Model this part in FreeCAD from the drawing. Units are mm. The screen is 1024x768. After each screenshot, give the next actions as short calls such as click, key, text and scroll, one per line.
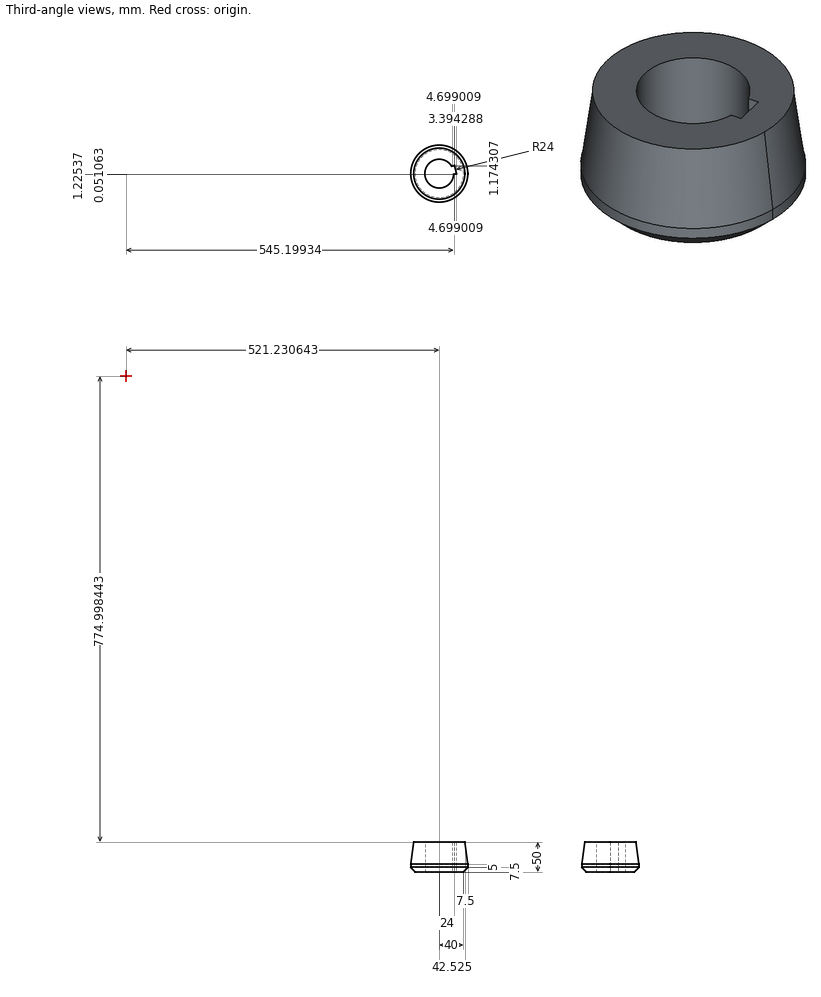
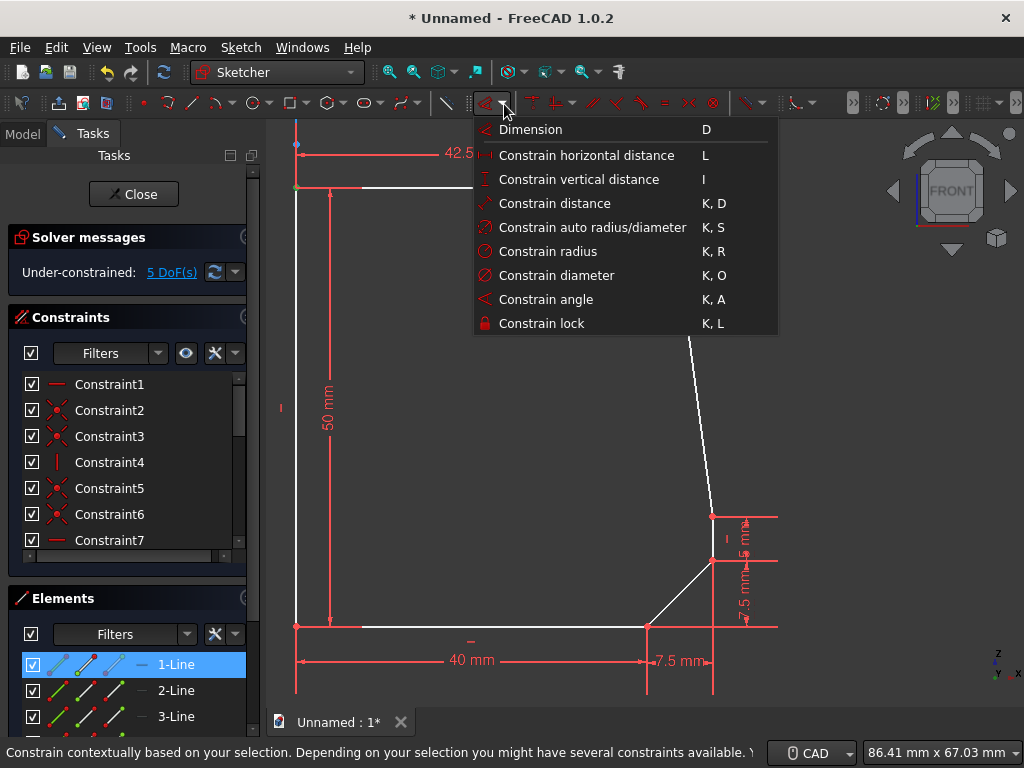
click(626, 155)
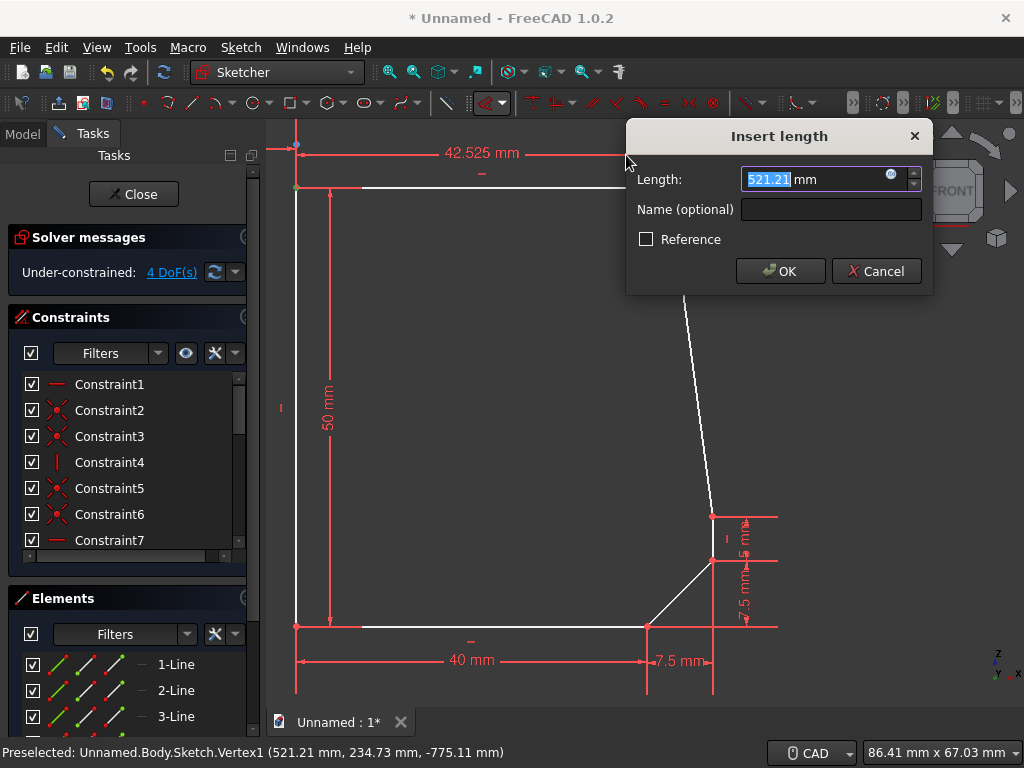
text(521.230643)
key(Return)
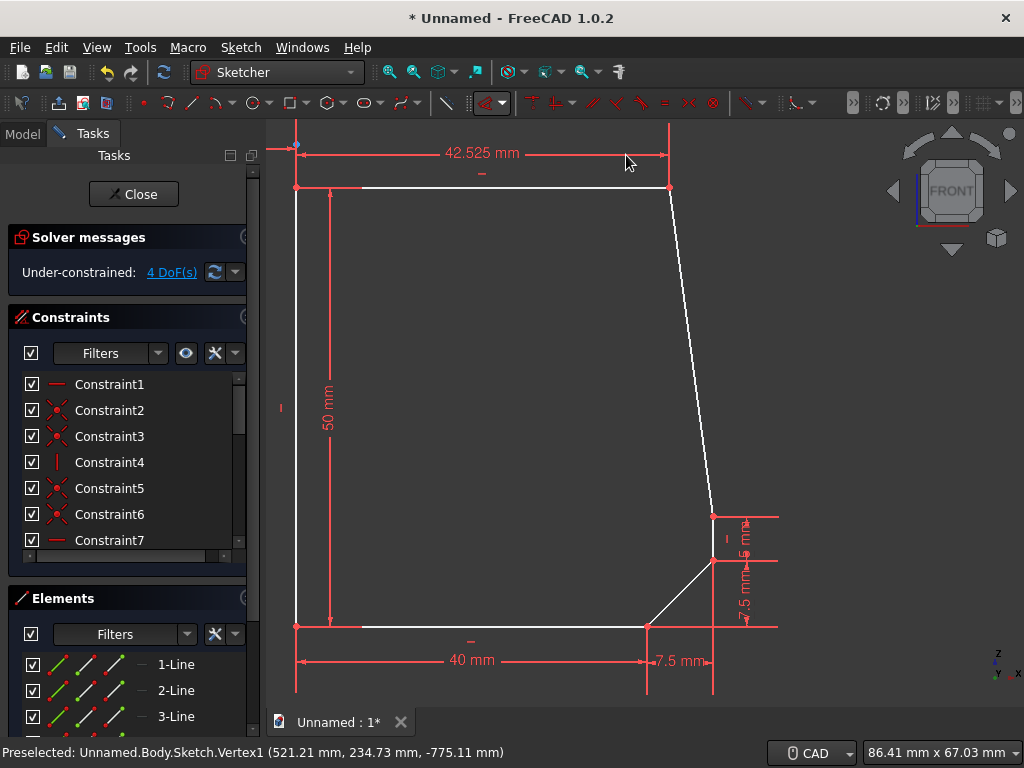
click(296, 188)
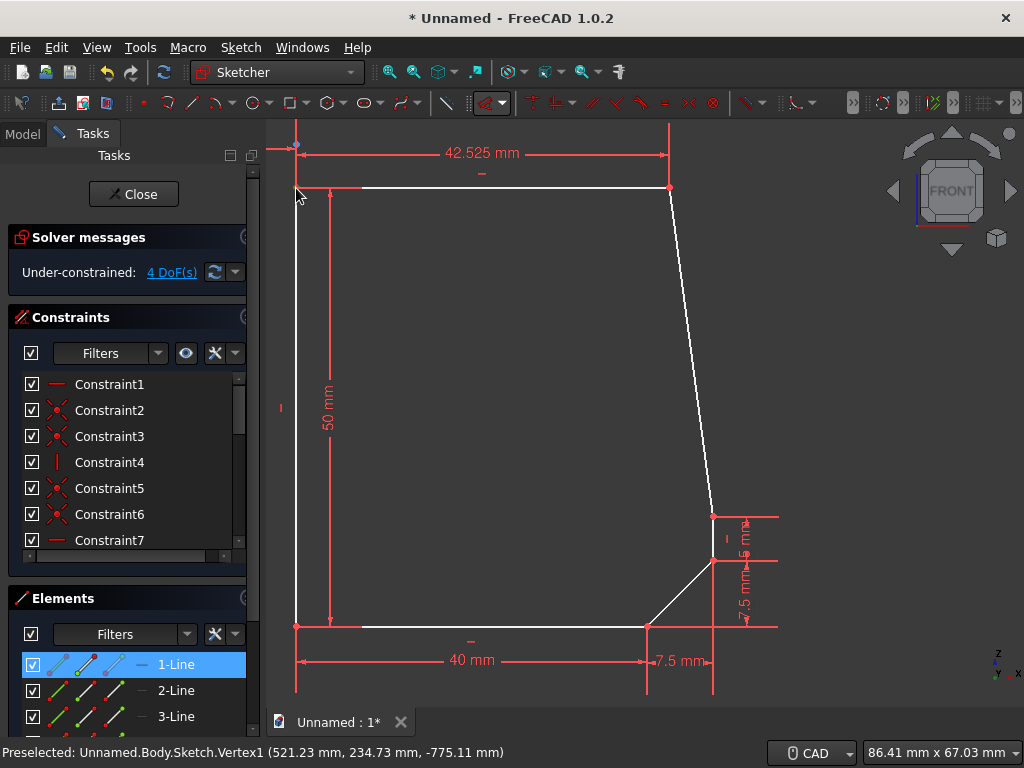
click(504, 104)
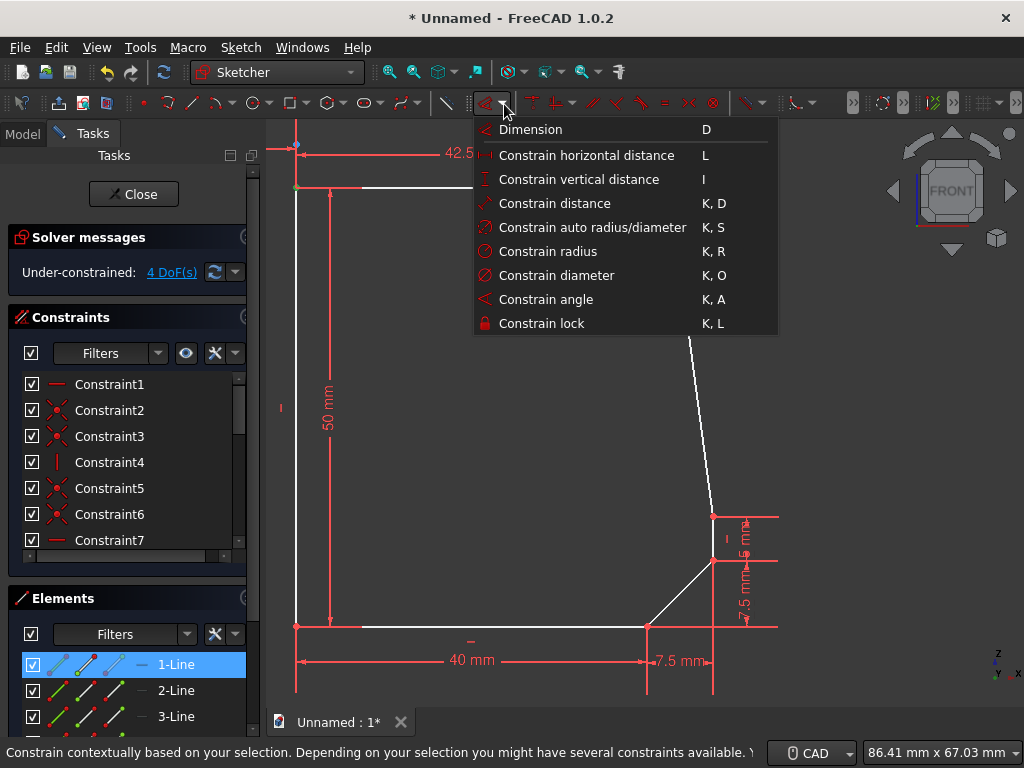
click(626, 179)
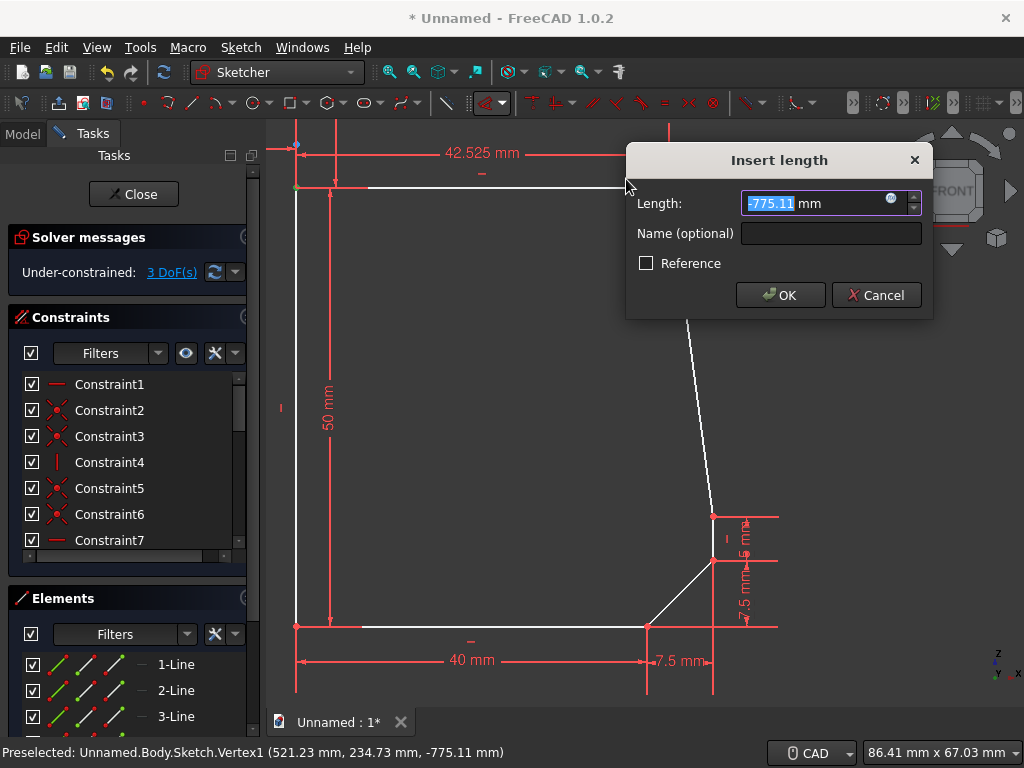
text(-774.998443)
key(Return)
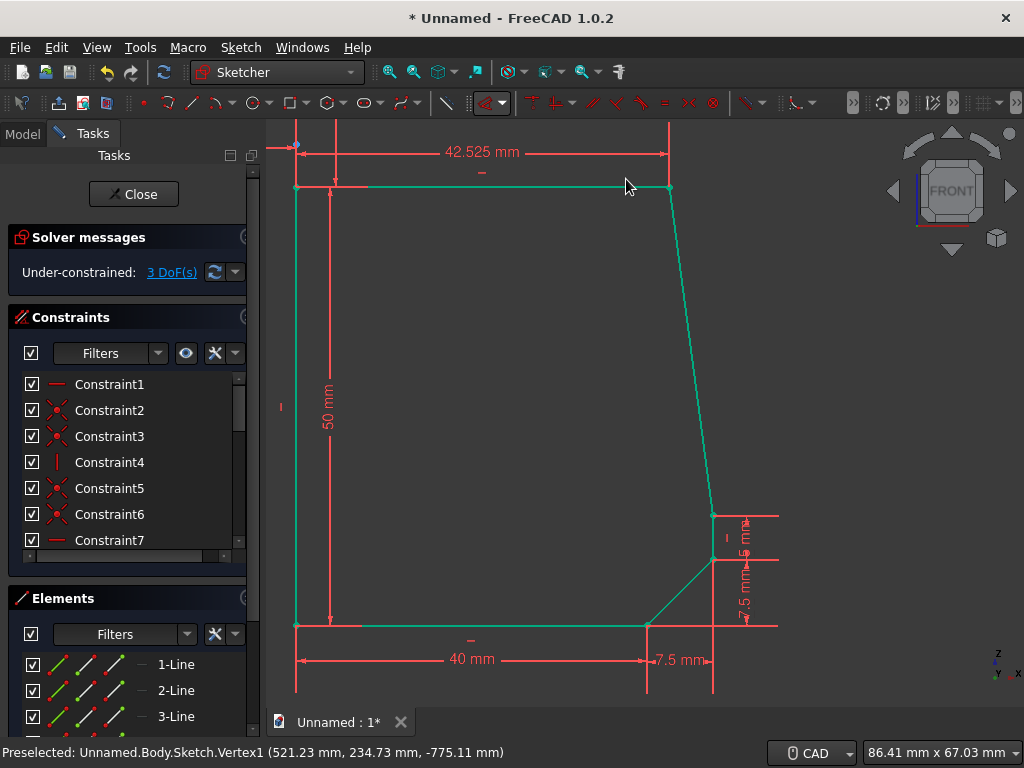
scroll(722, 605, down, 2)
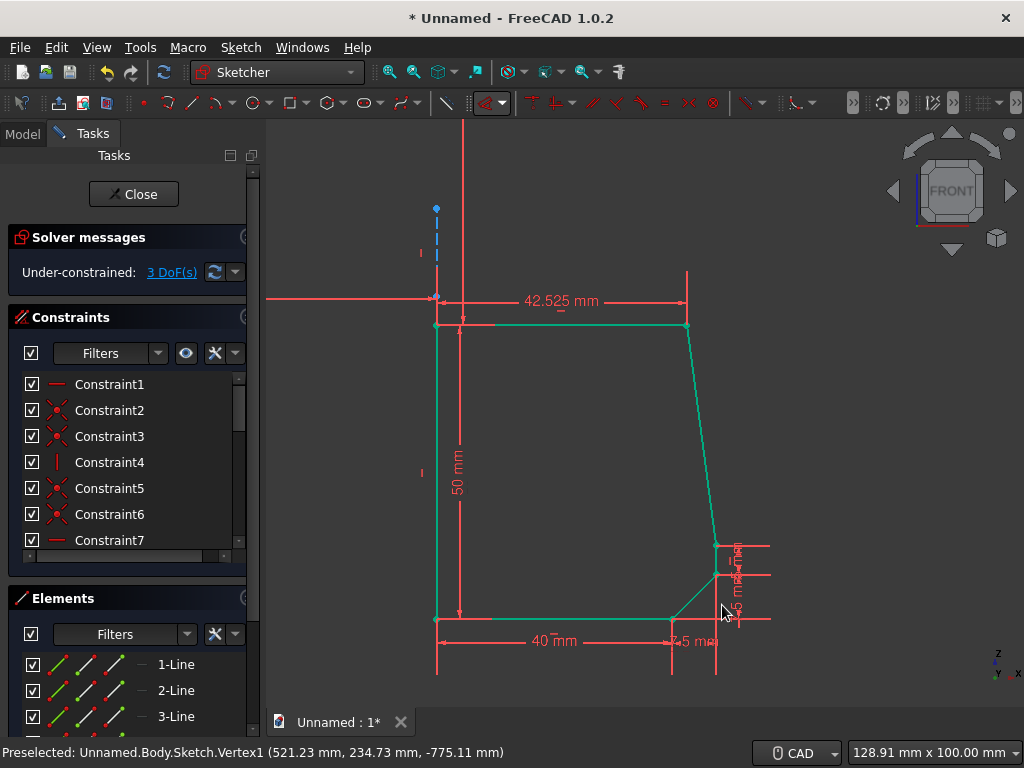
click(437, 297)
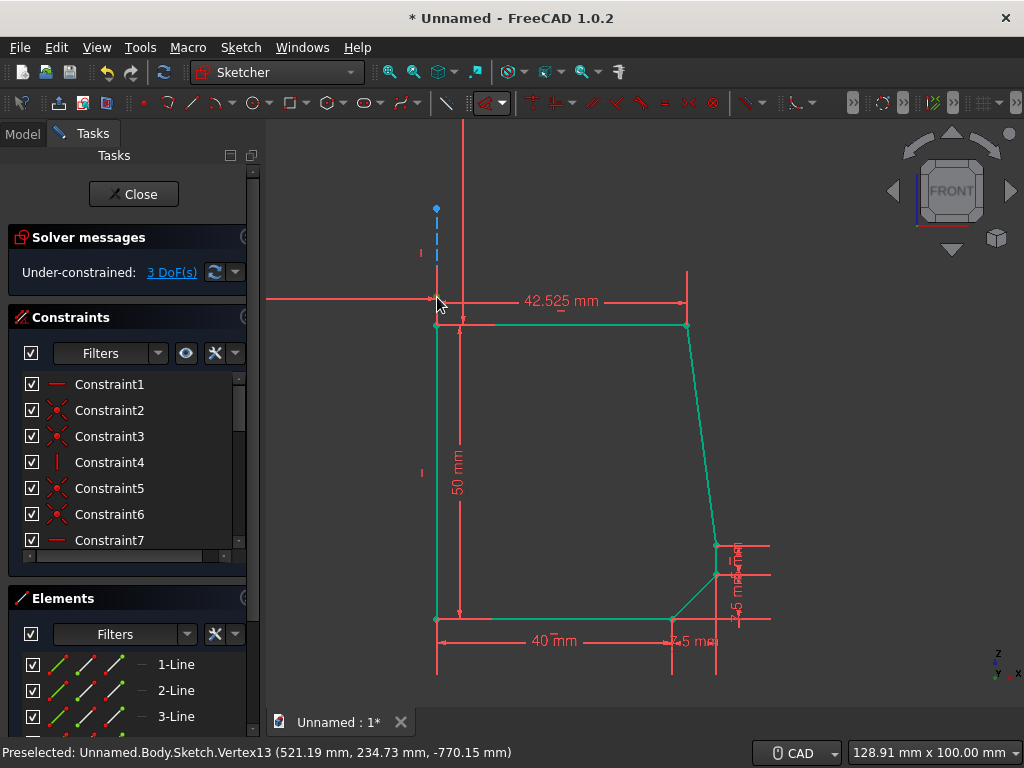
click(504, 104)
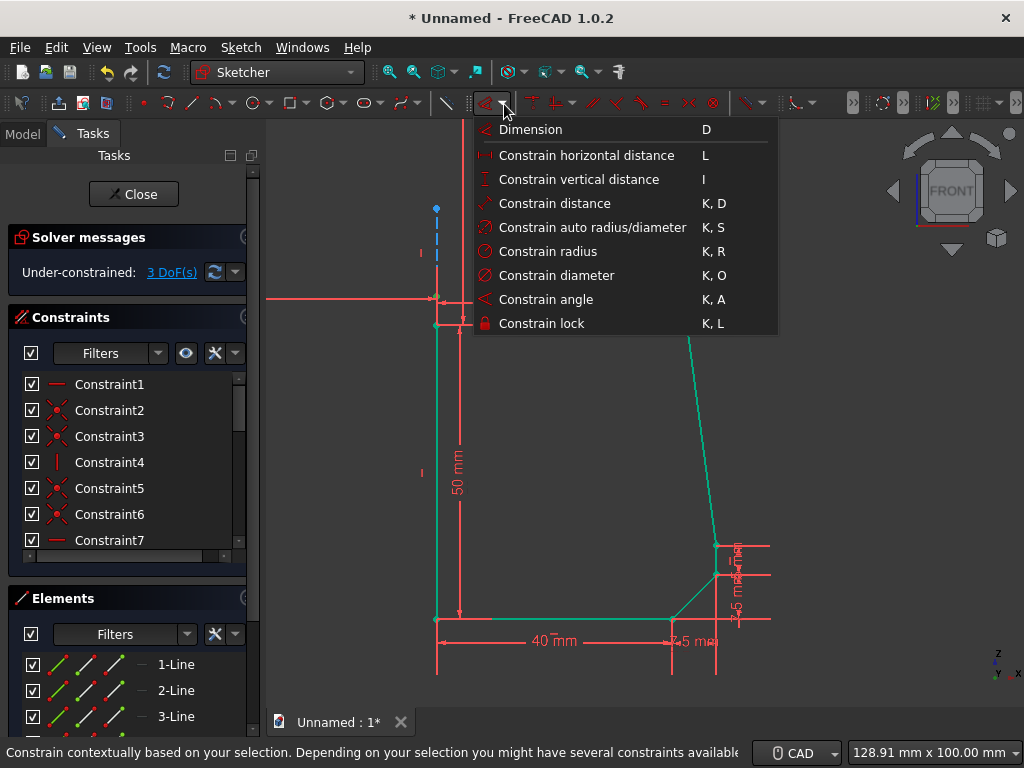
click(626, 155)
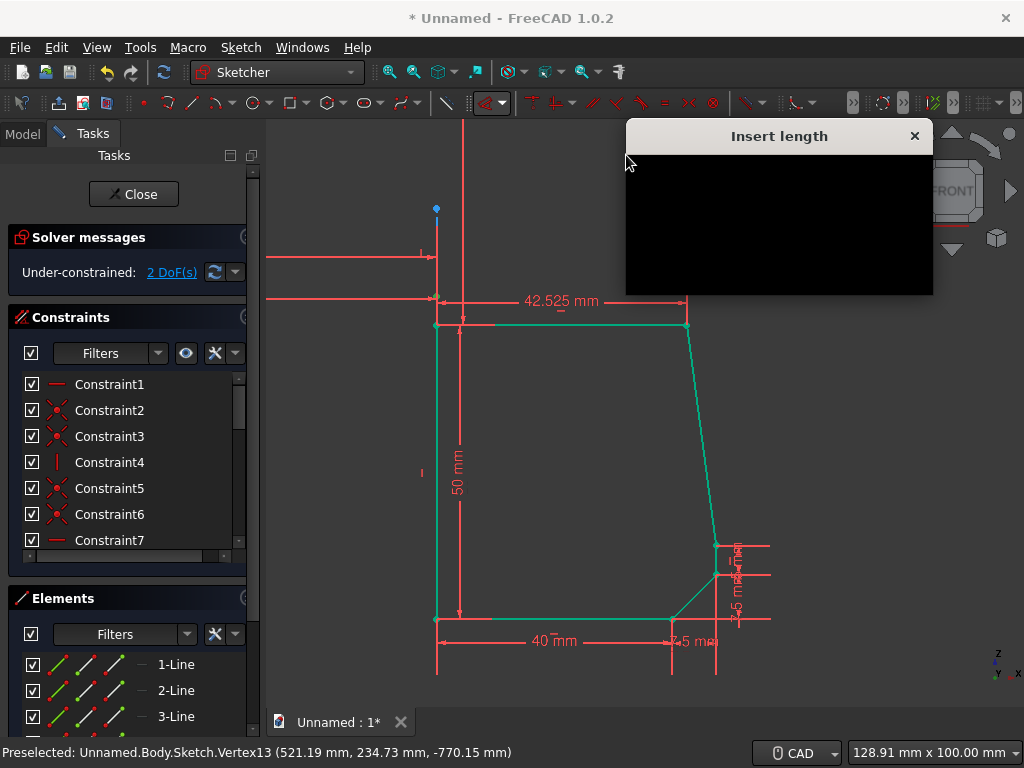
text(521.230643)
key(Return)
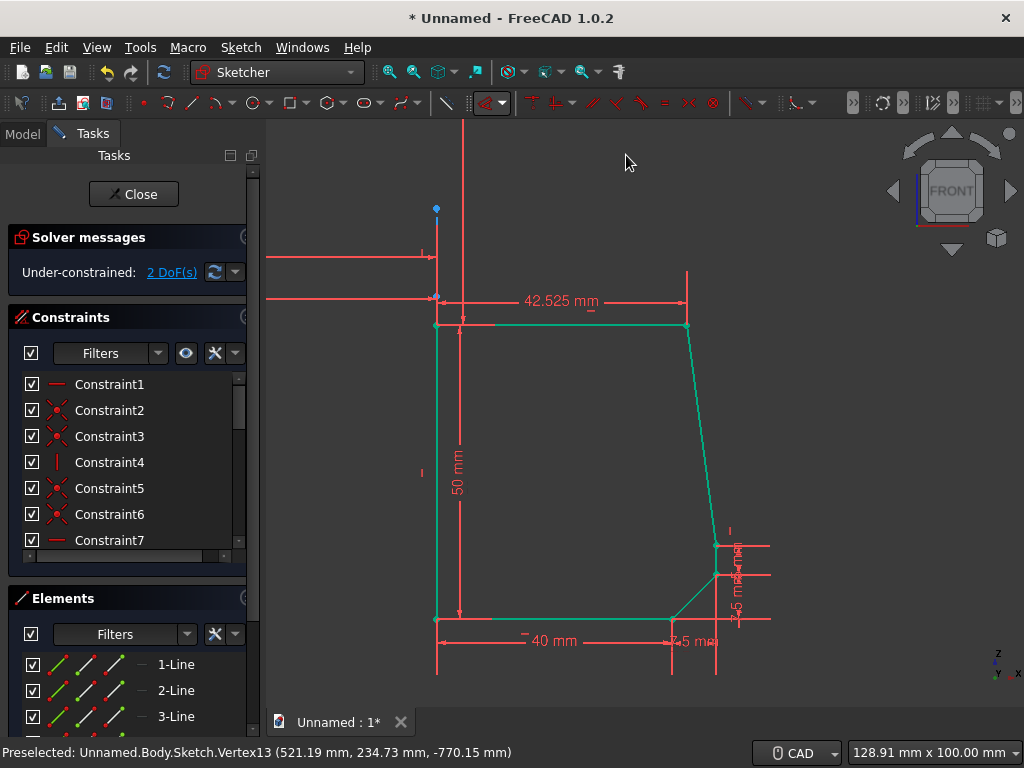
click(134, 194)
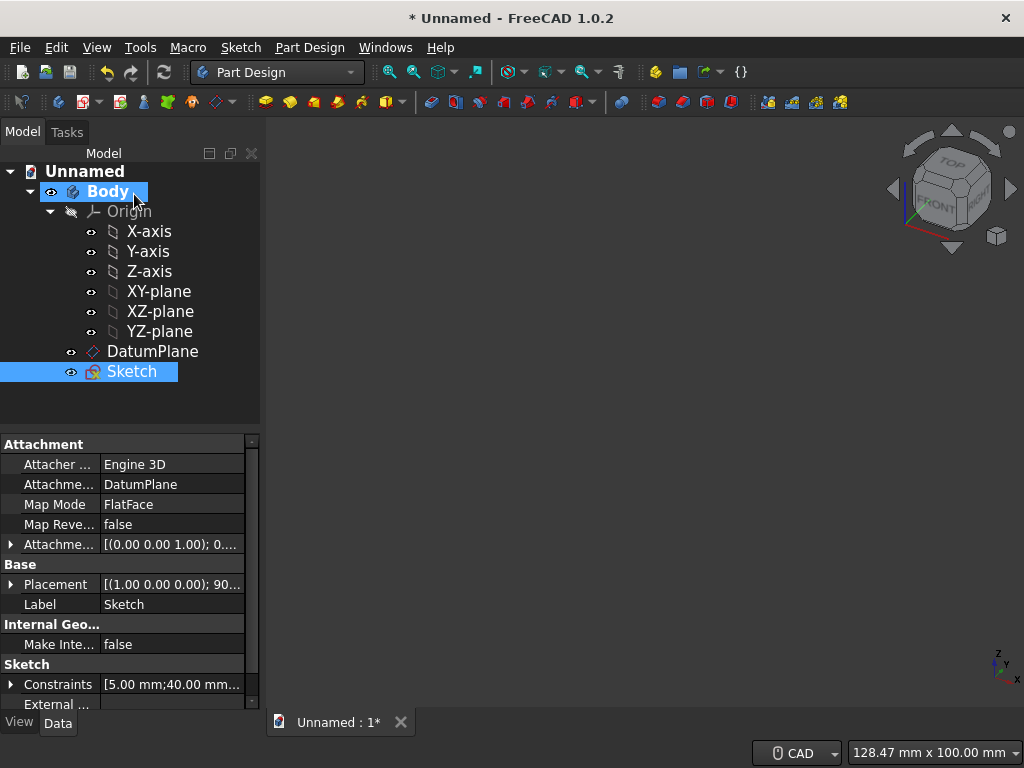
click(290, 102)